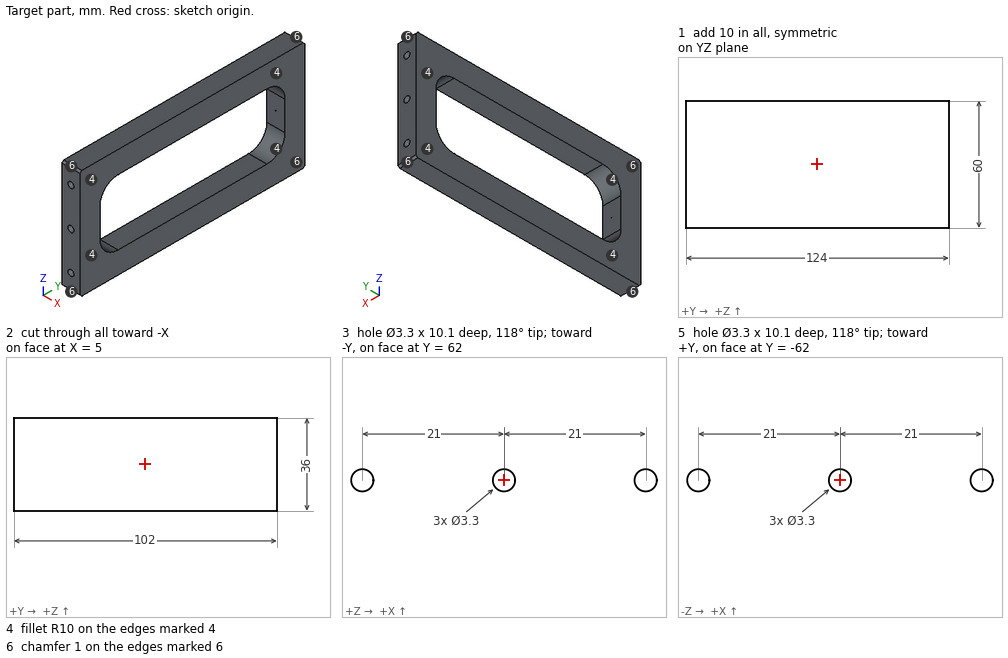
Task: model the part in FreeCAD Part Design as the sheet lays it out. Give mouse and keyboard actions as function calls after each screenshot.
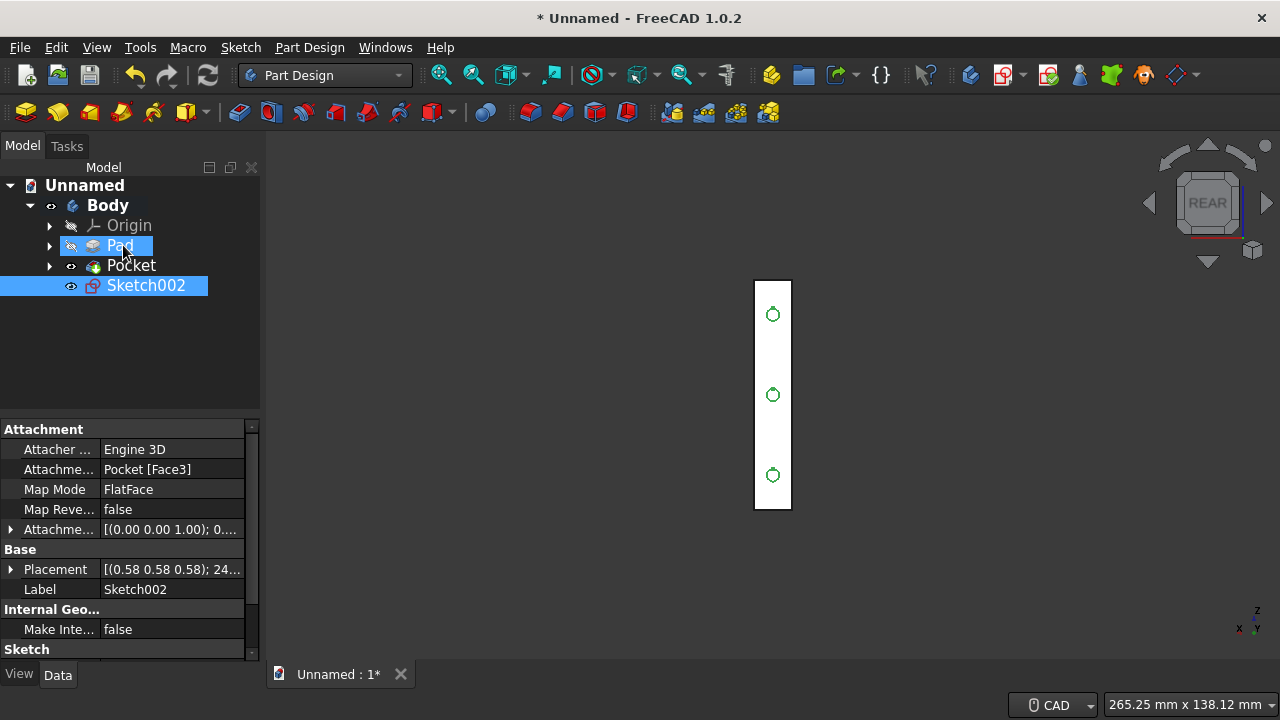
click(272, 112)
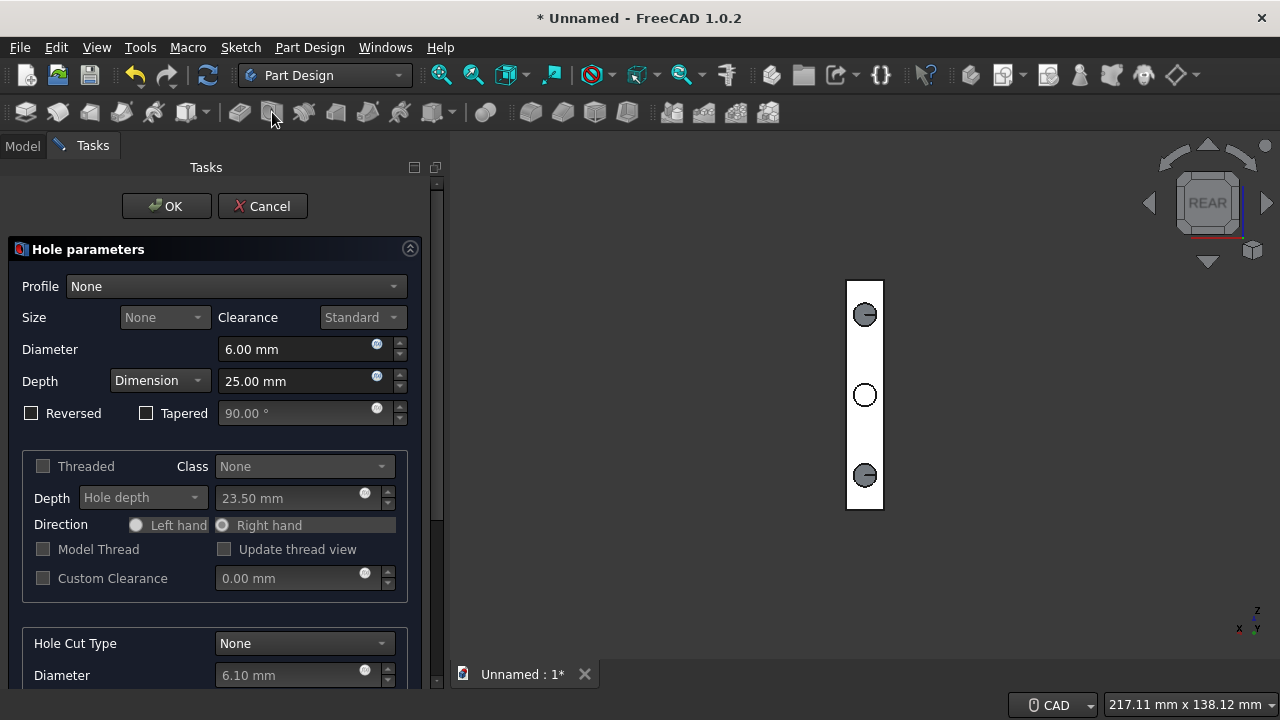
triple_click(305, 349)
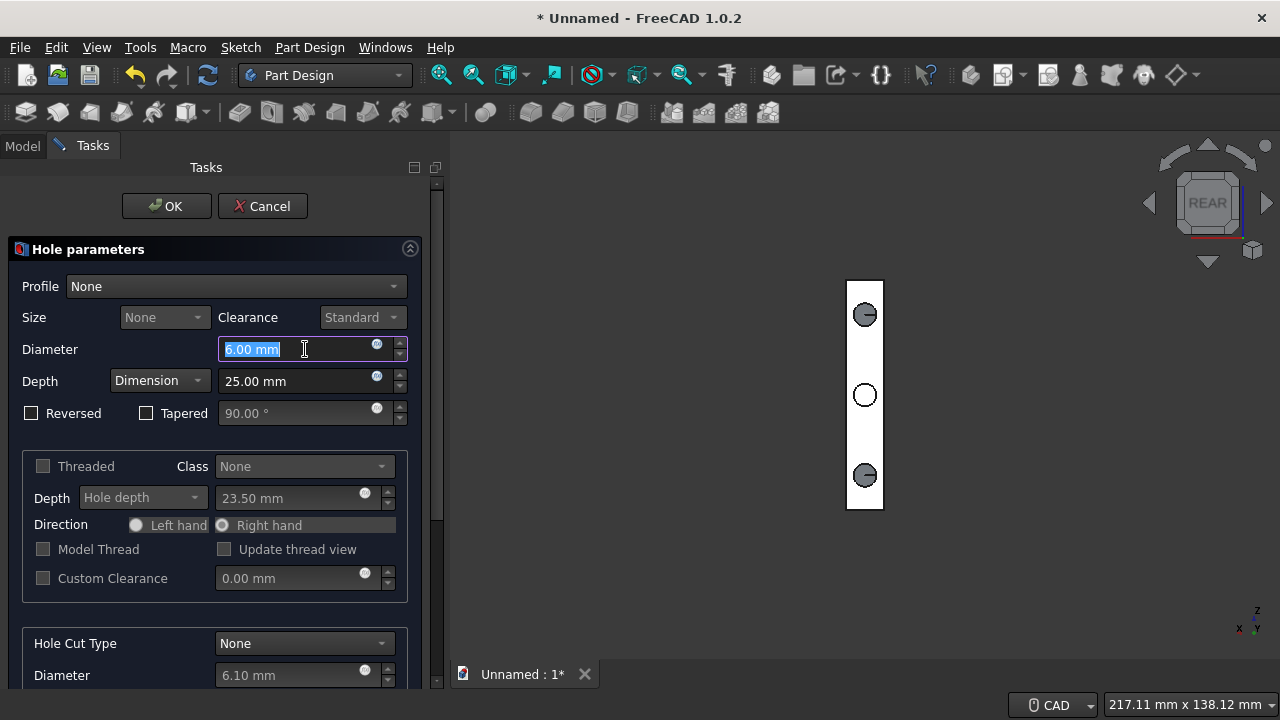
text(3.3)
key(Tab)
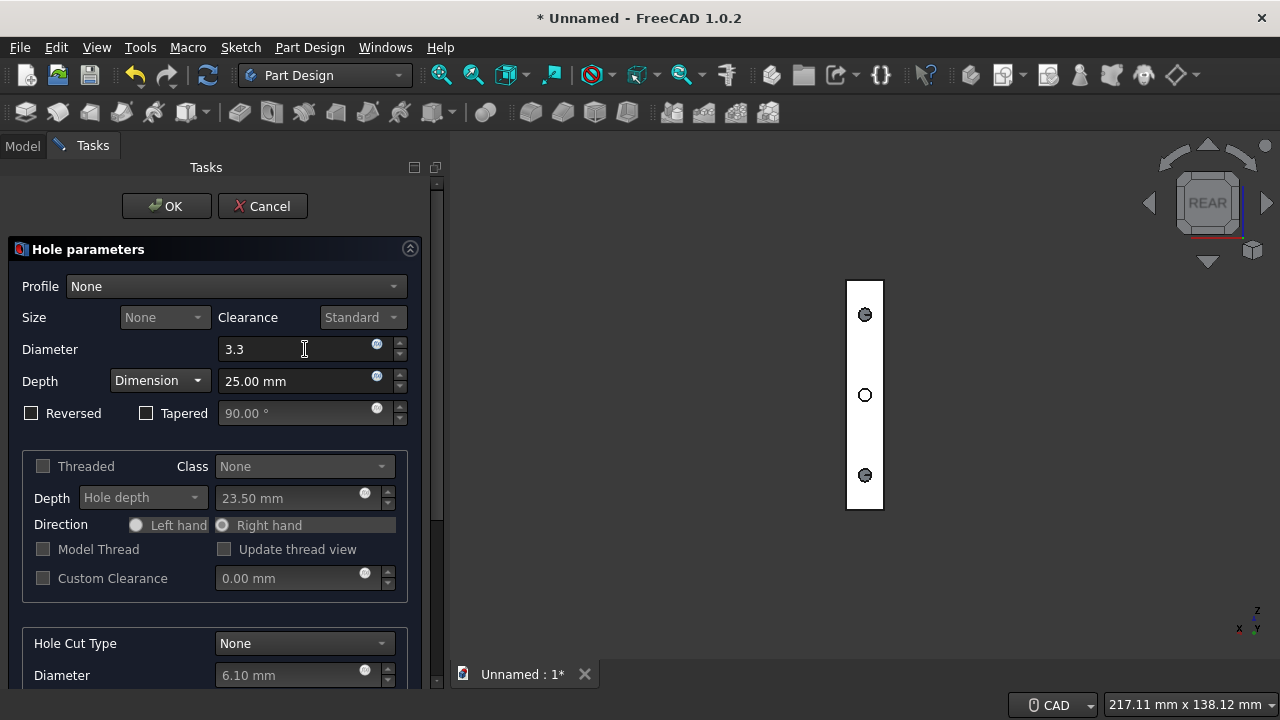
triple_click(305, 381)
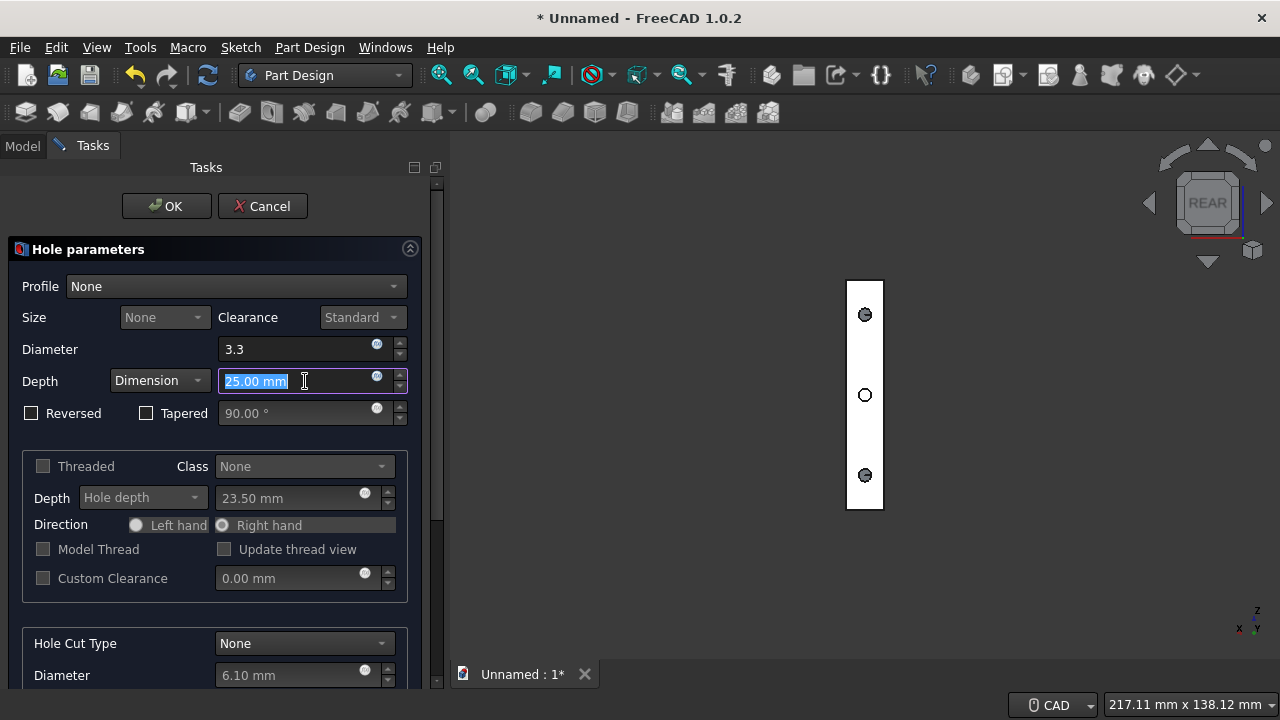
text(10.1)
key(Tab)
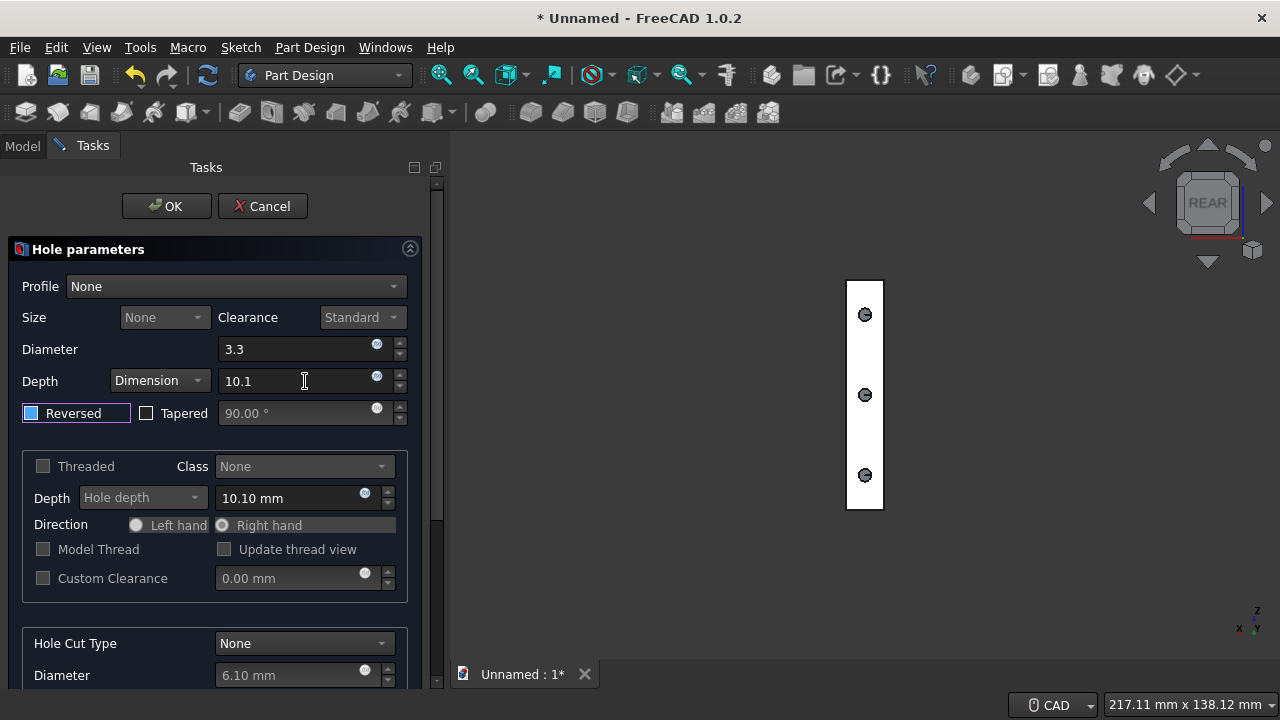
click(167, 206)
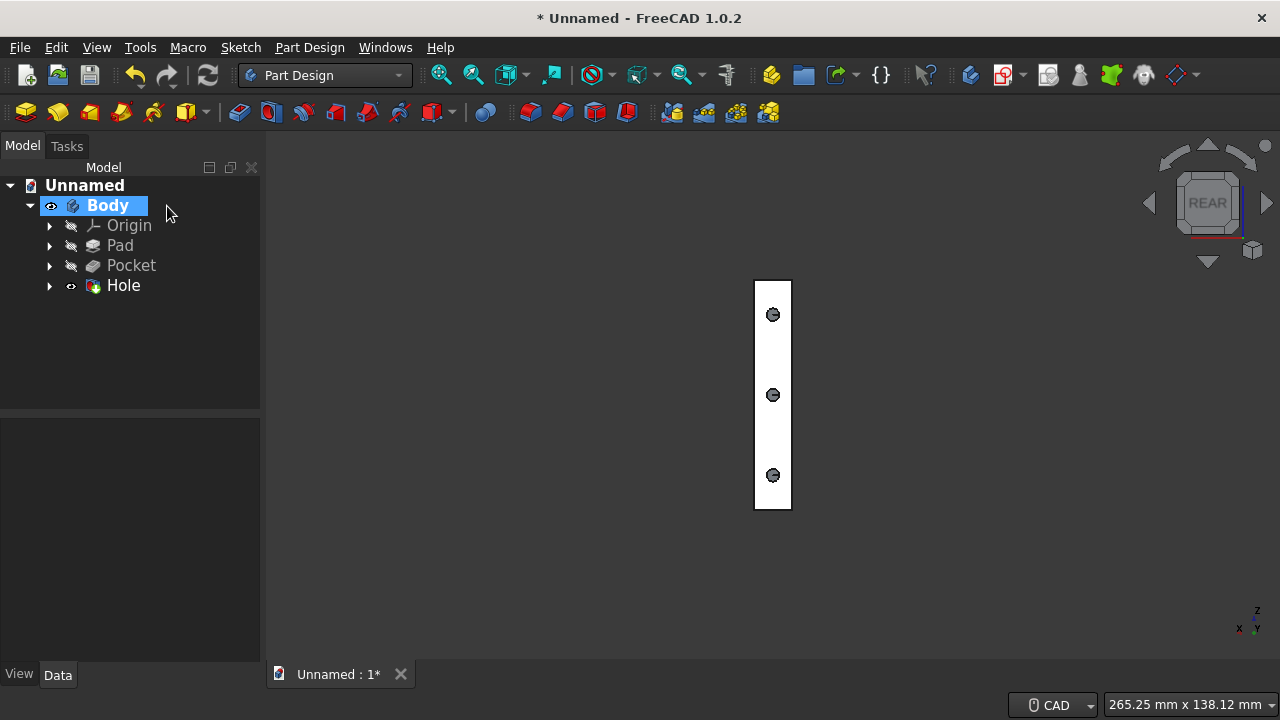
click(442, 76)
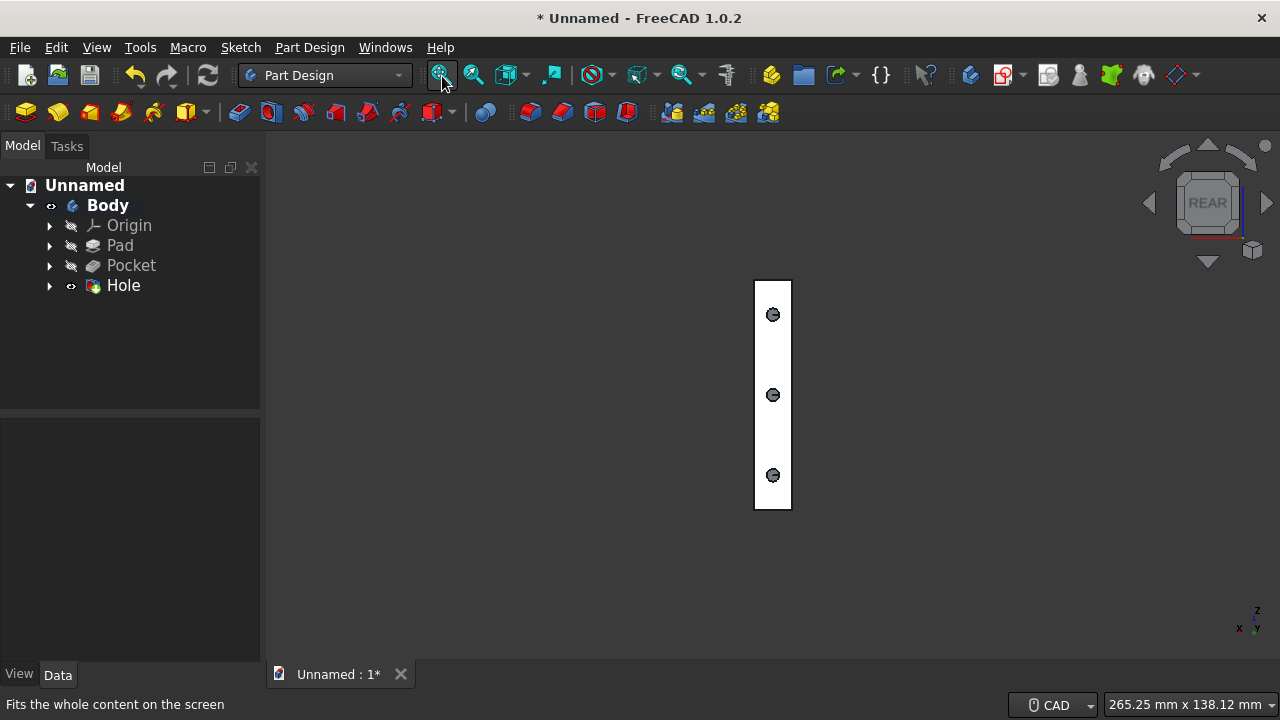
key(0)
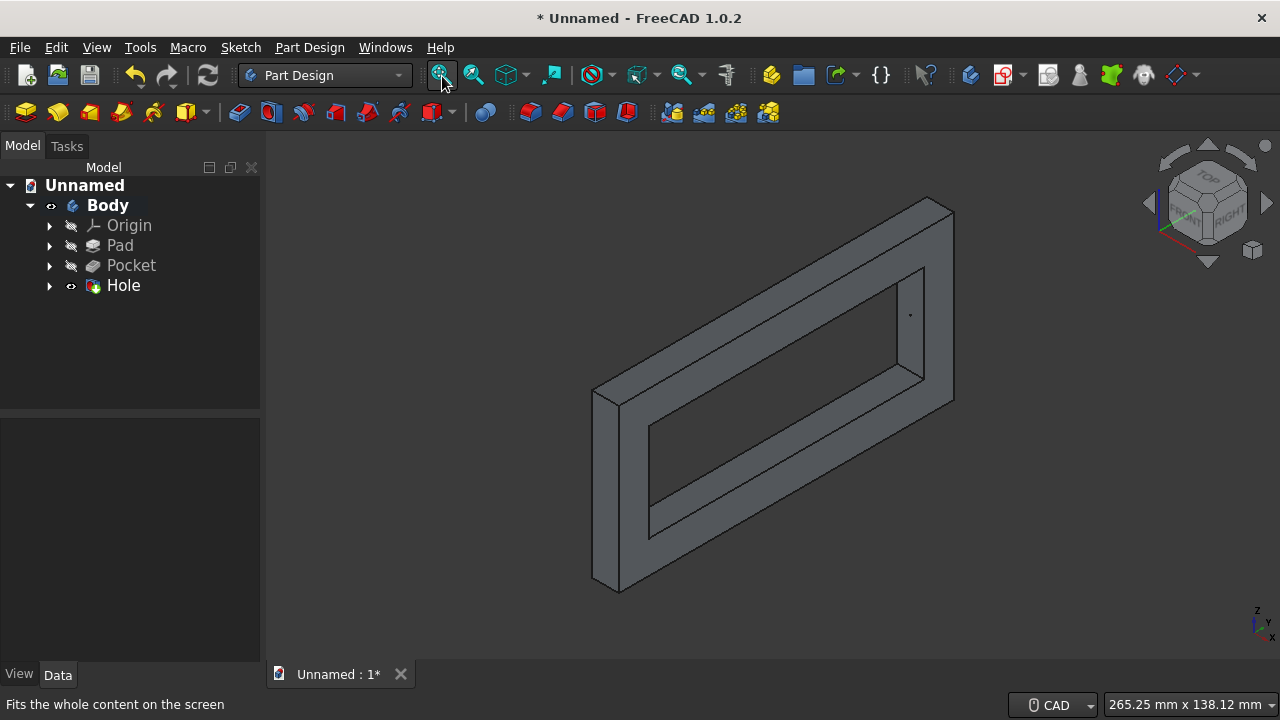
key(2)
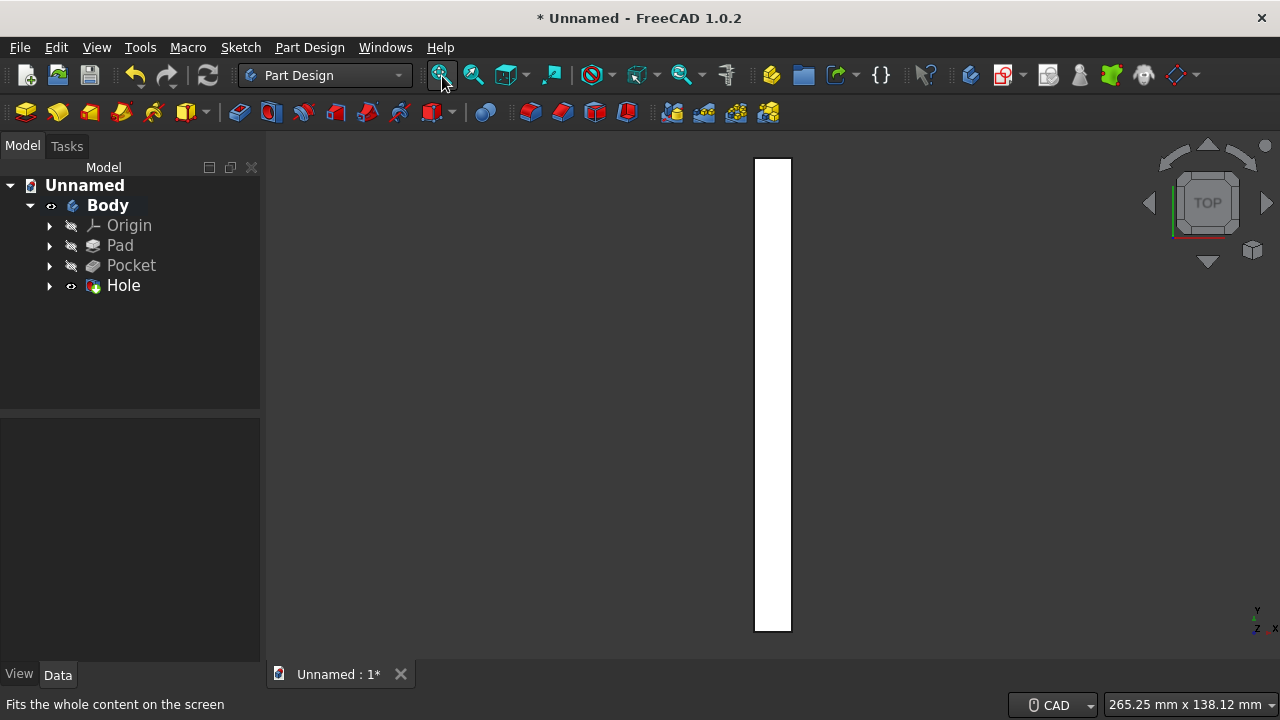
key(1)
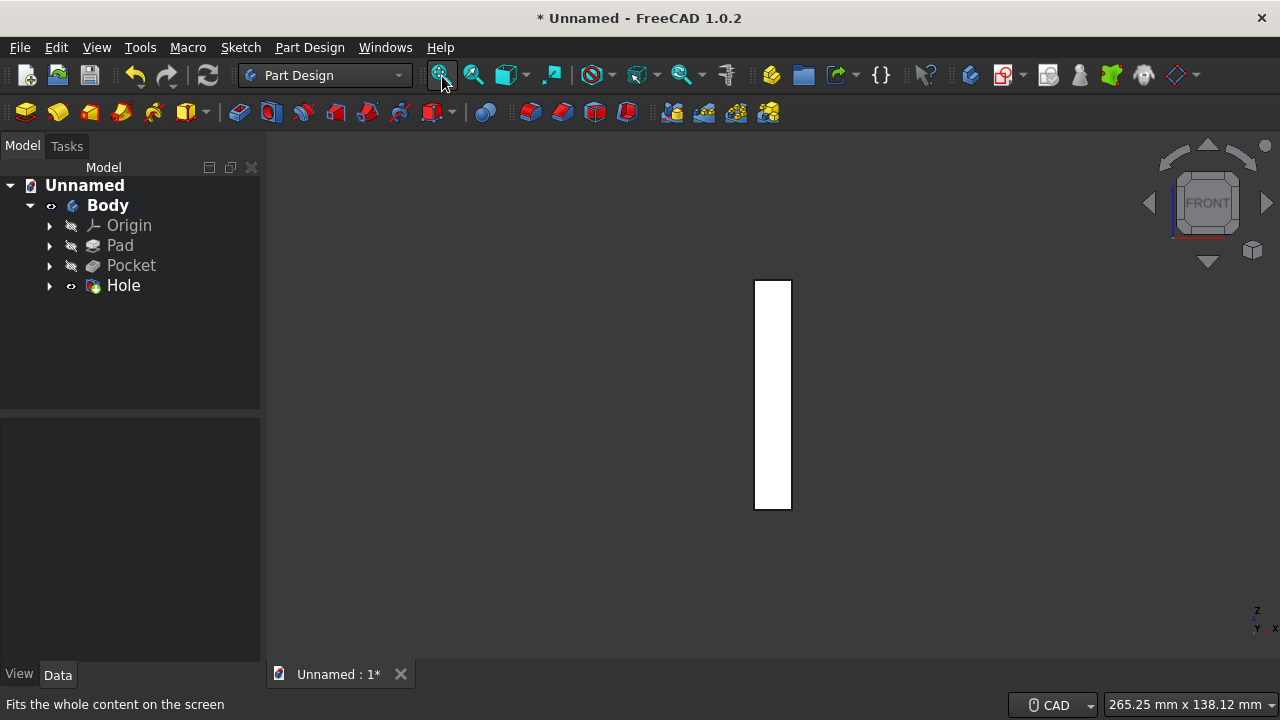
click(442, 76)